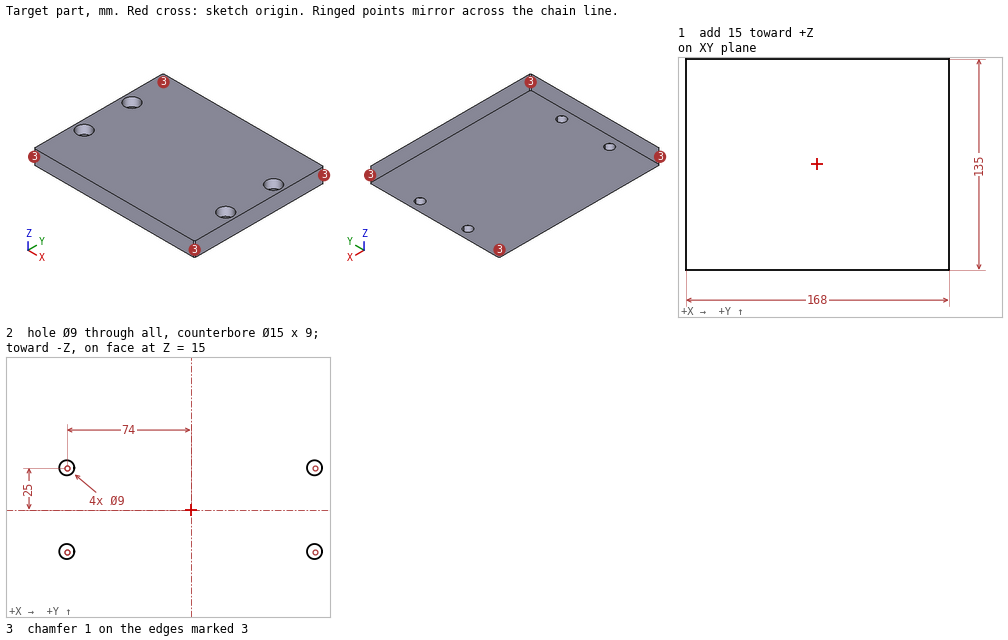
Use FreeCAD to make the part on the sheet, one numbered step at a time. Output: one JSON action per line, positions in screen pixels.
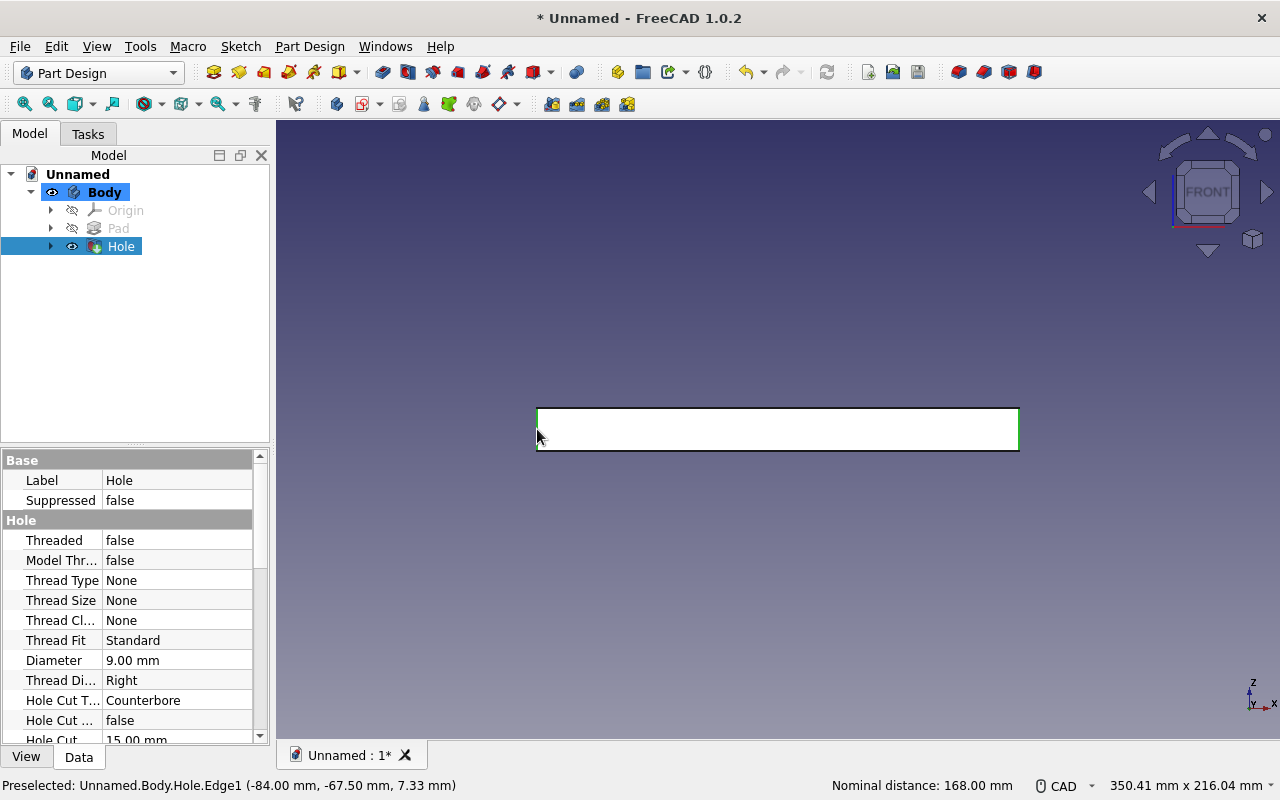
{"action": "key", "text": "3"}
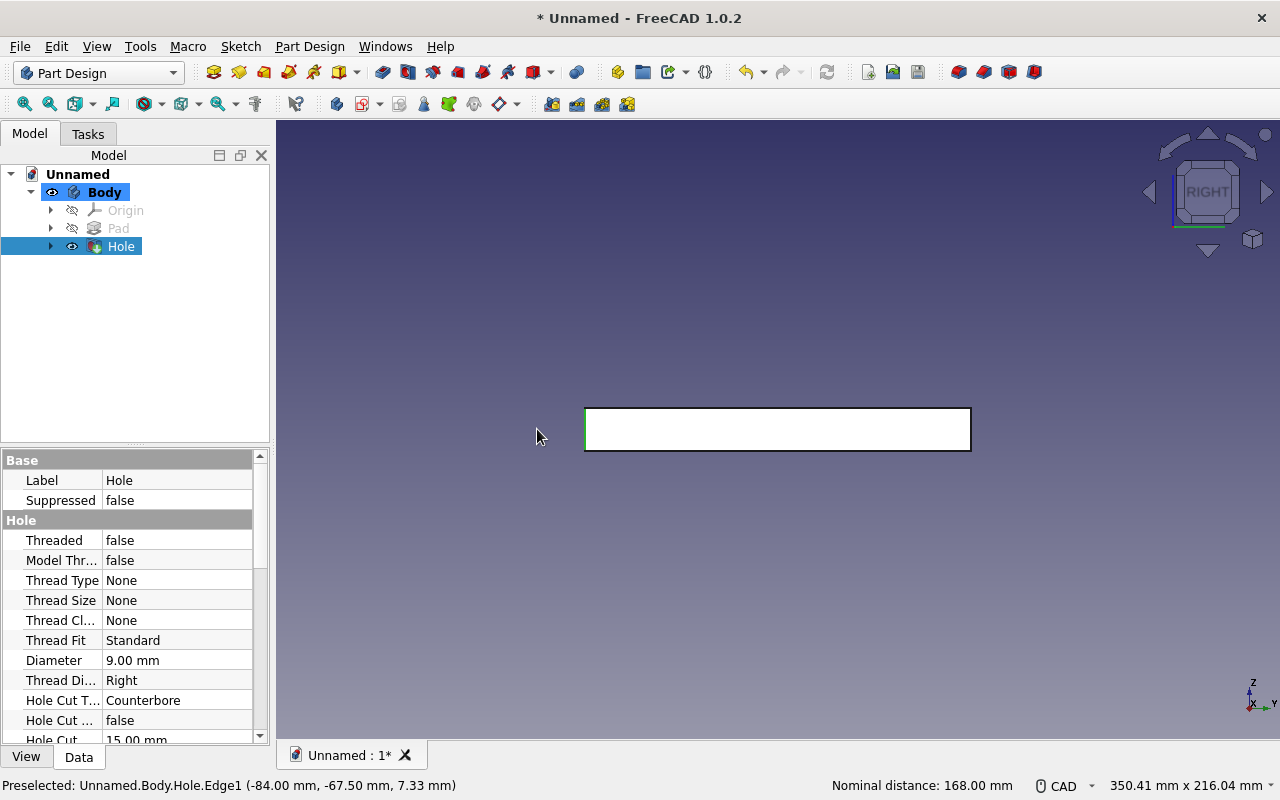
{"action": "left_click", "coordinate": [25, 104]}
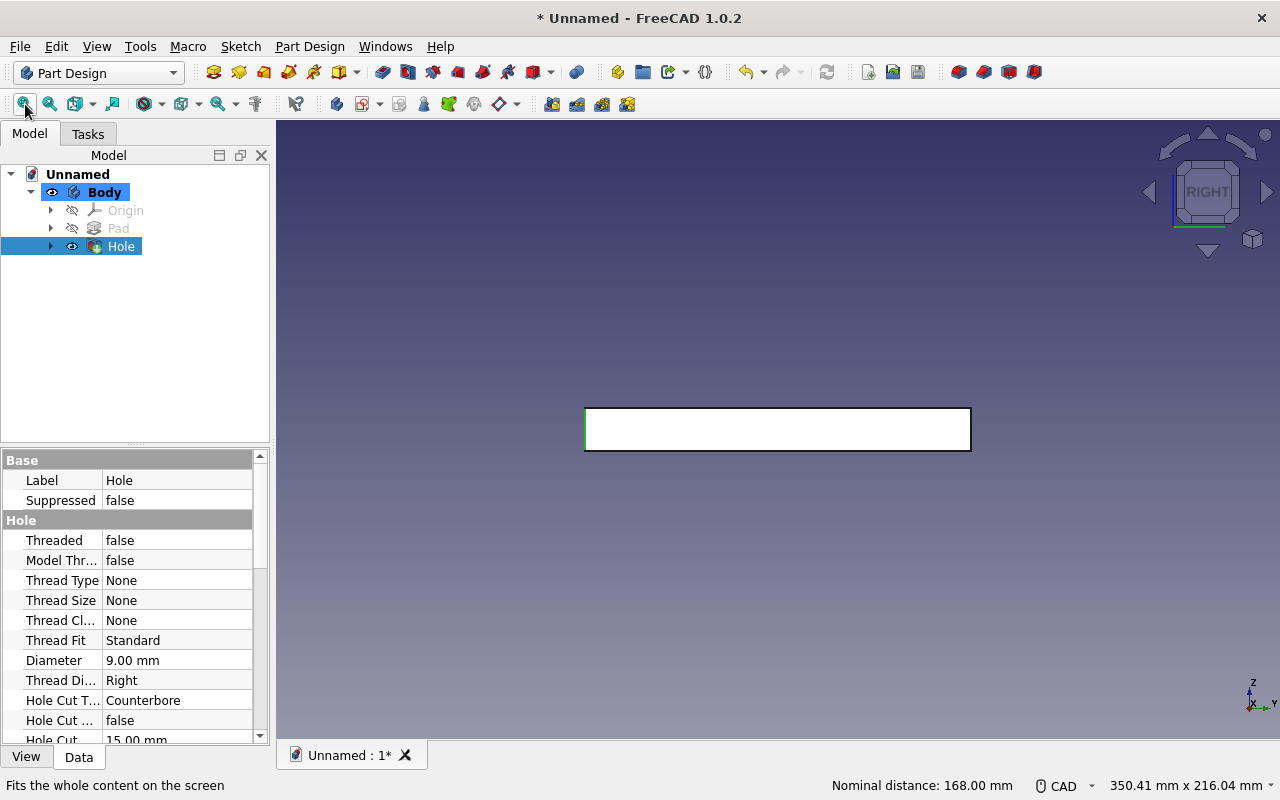
{"action": "left_click", "coordinate": [971, 428], "text": "ctrl"}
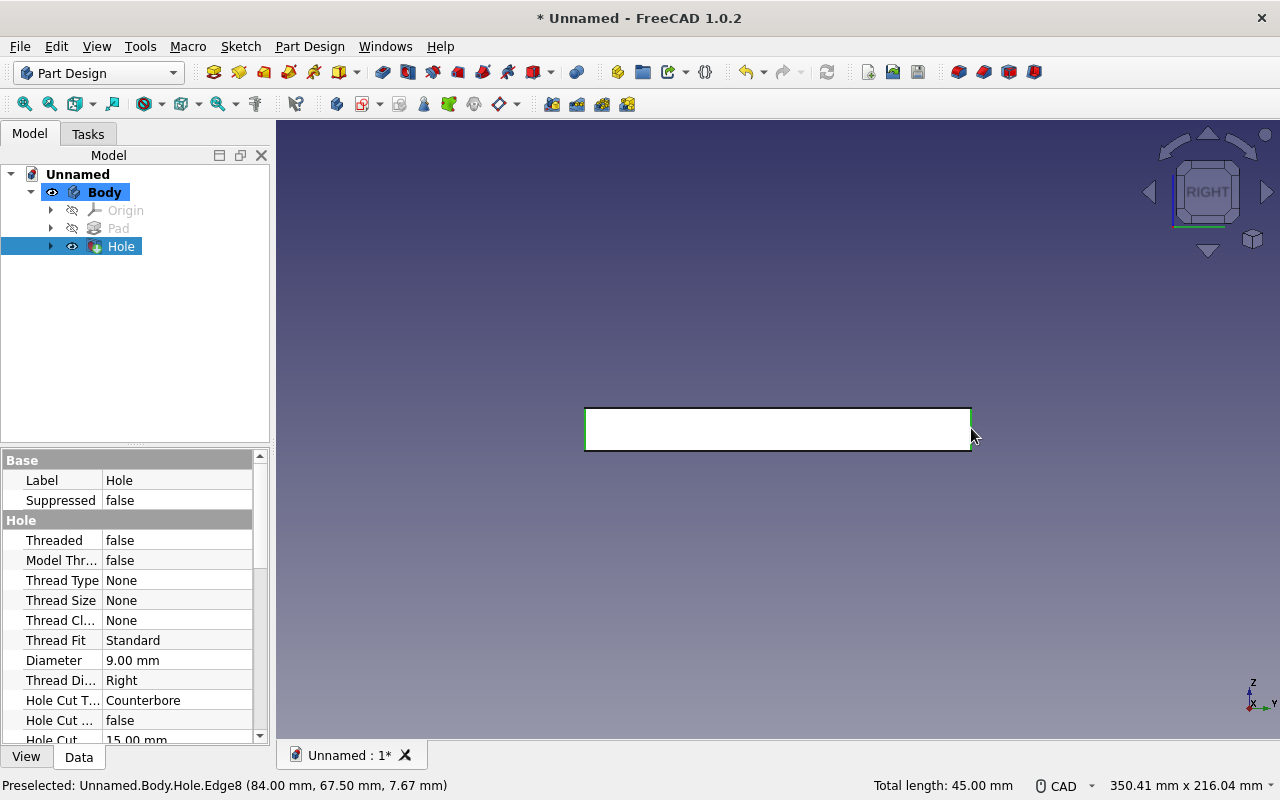
{"action": "key", "text": "5"}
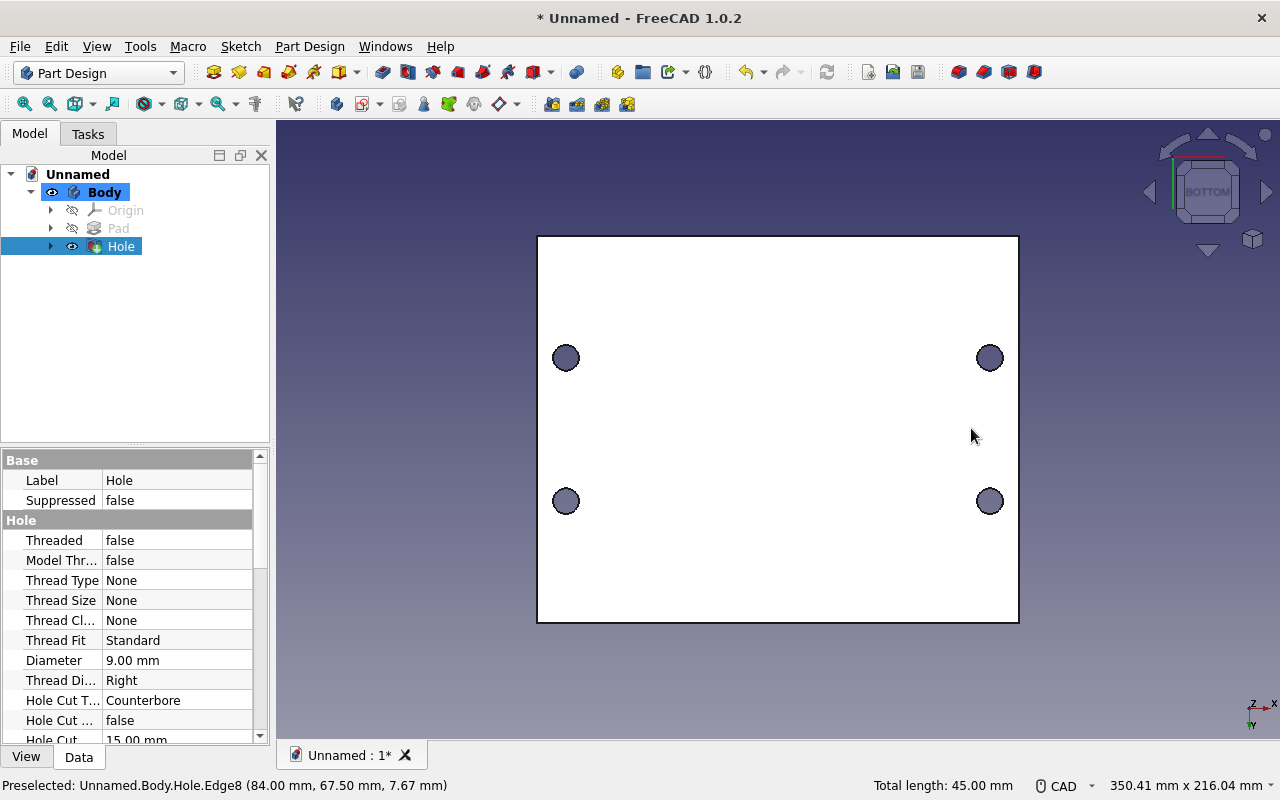
{"action": "key", "text": "4"}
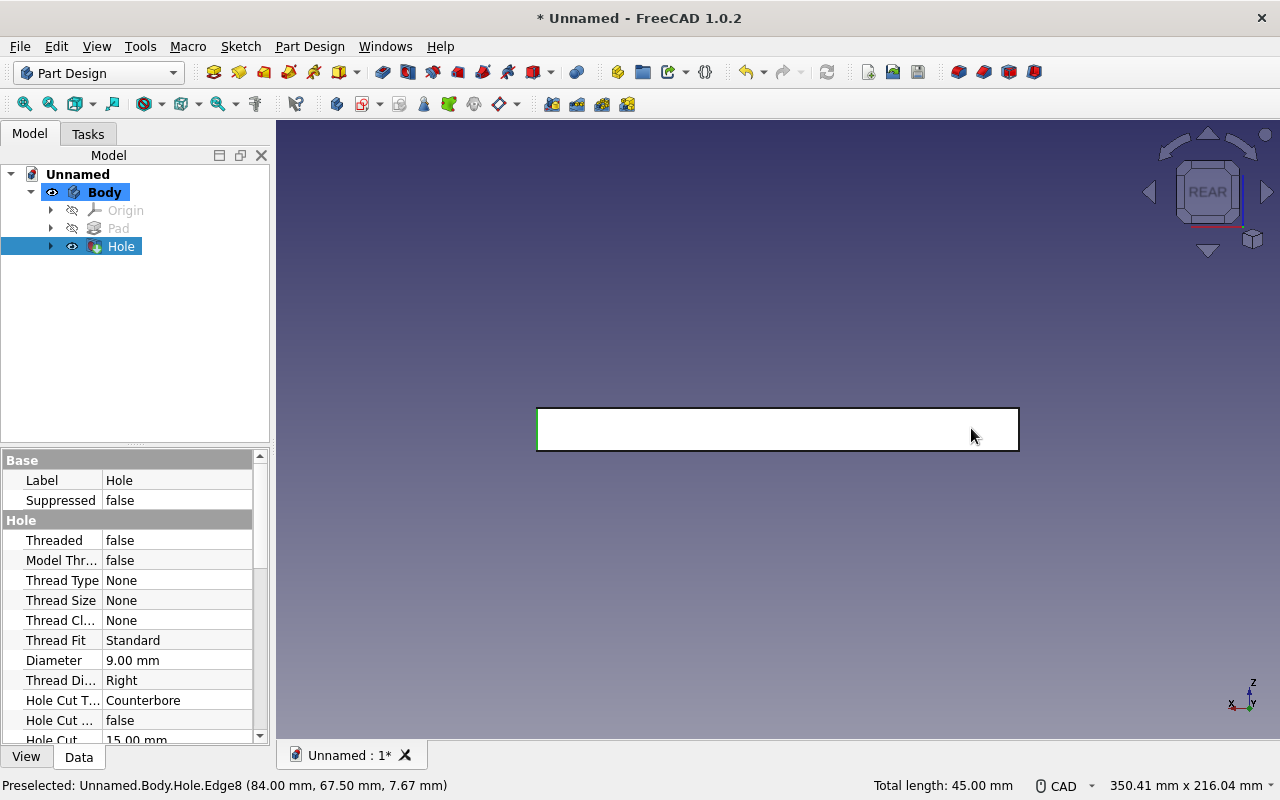
{"action": "left_click", "coordinate": [1019, 429], "text": "ctrl"}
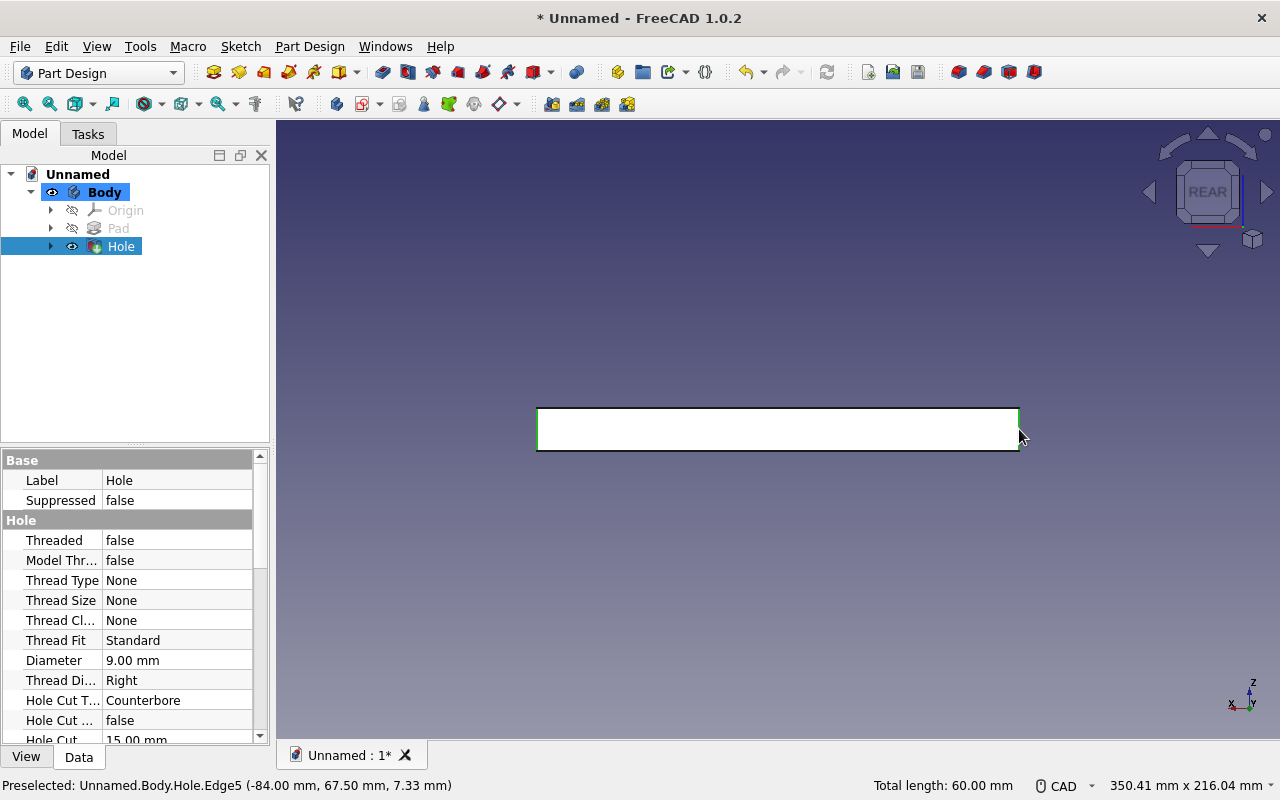
{"action": "left_click", "coordinate": [984, 72]}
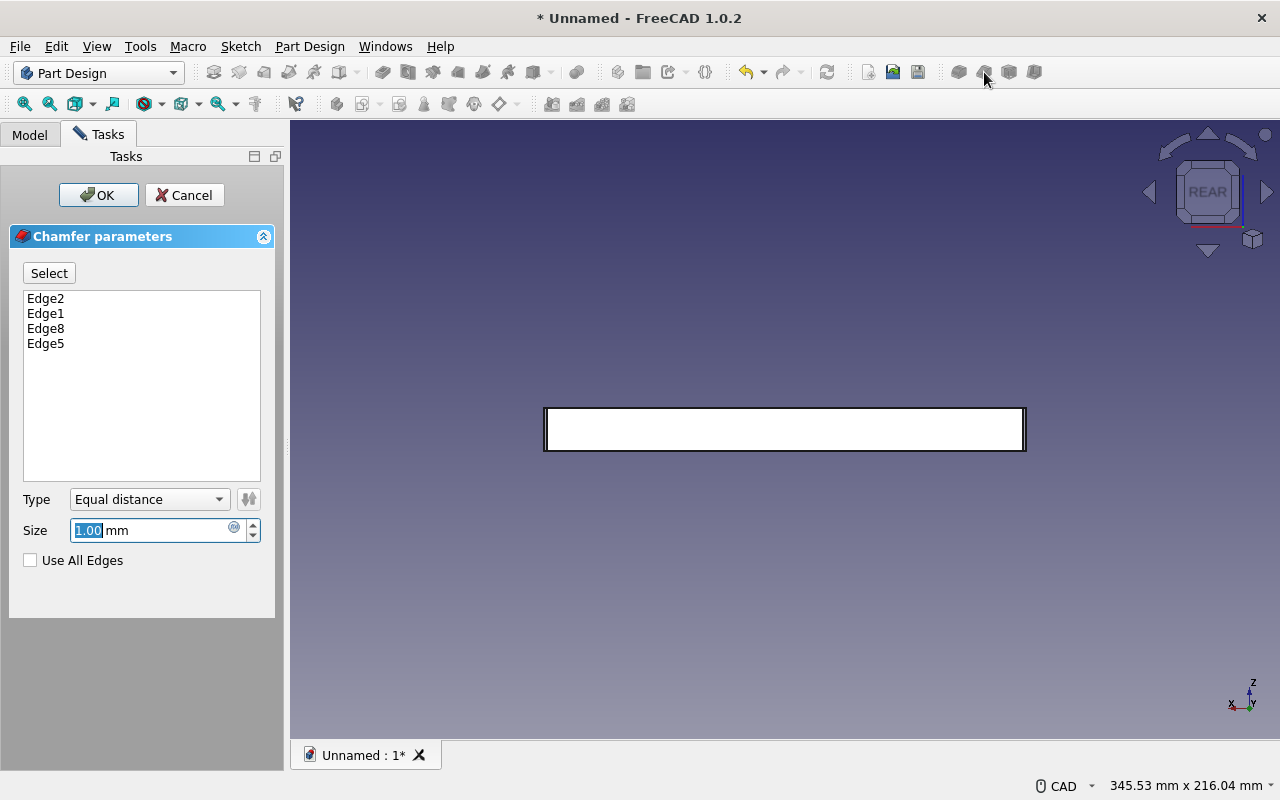
{"action": "type", "text": "1"}
{"action": "key", "text": "Tab"}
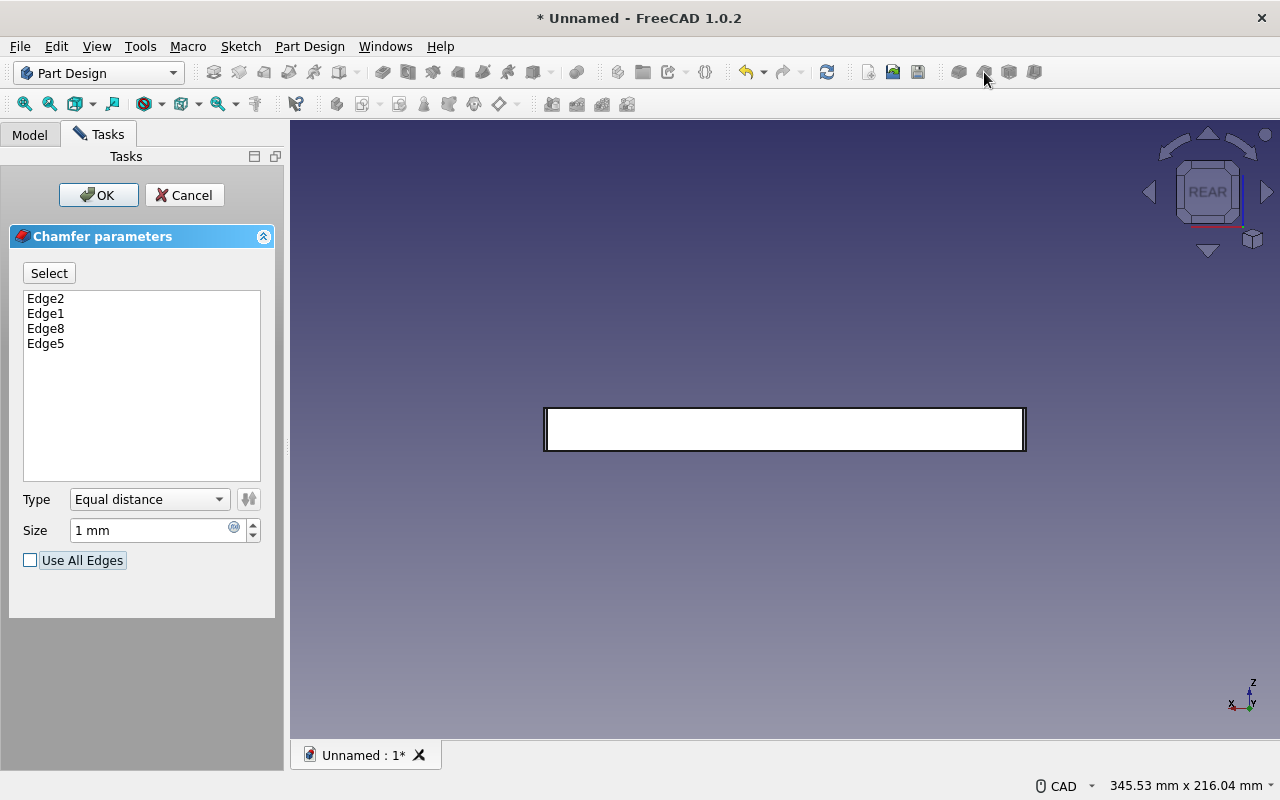
{"action": "left_click", "coordinate": [99, 195]}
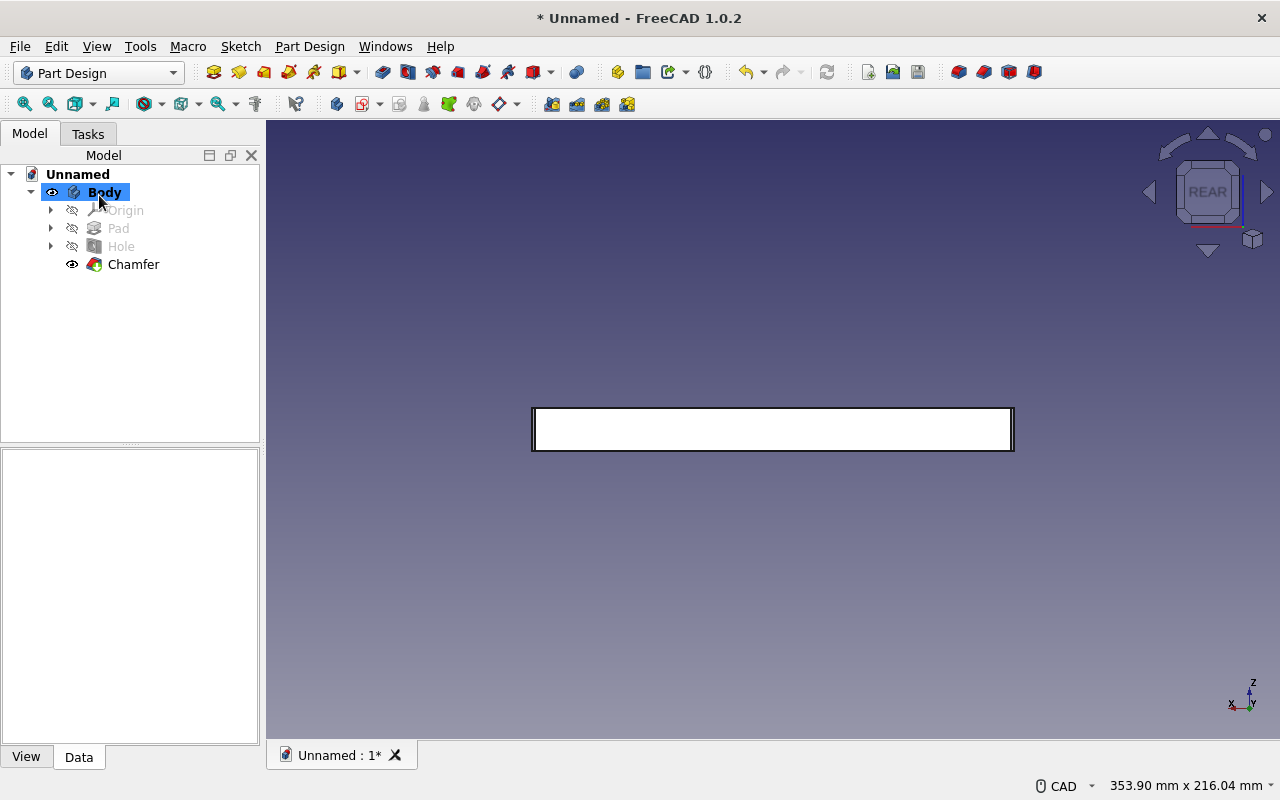
{"action": "key", "text": "0"}